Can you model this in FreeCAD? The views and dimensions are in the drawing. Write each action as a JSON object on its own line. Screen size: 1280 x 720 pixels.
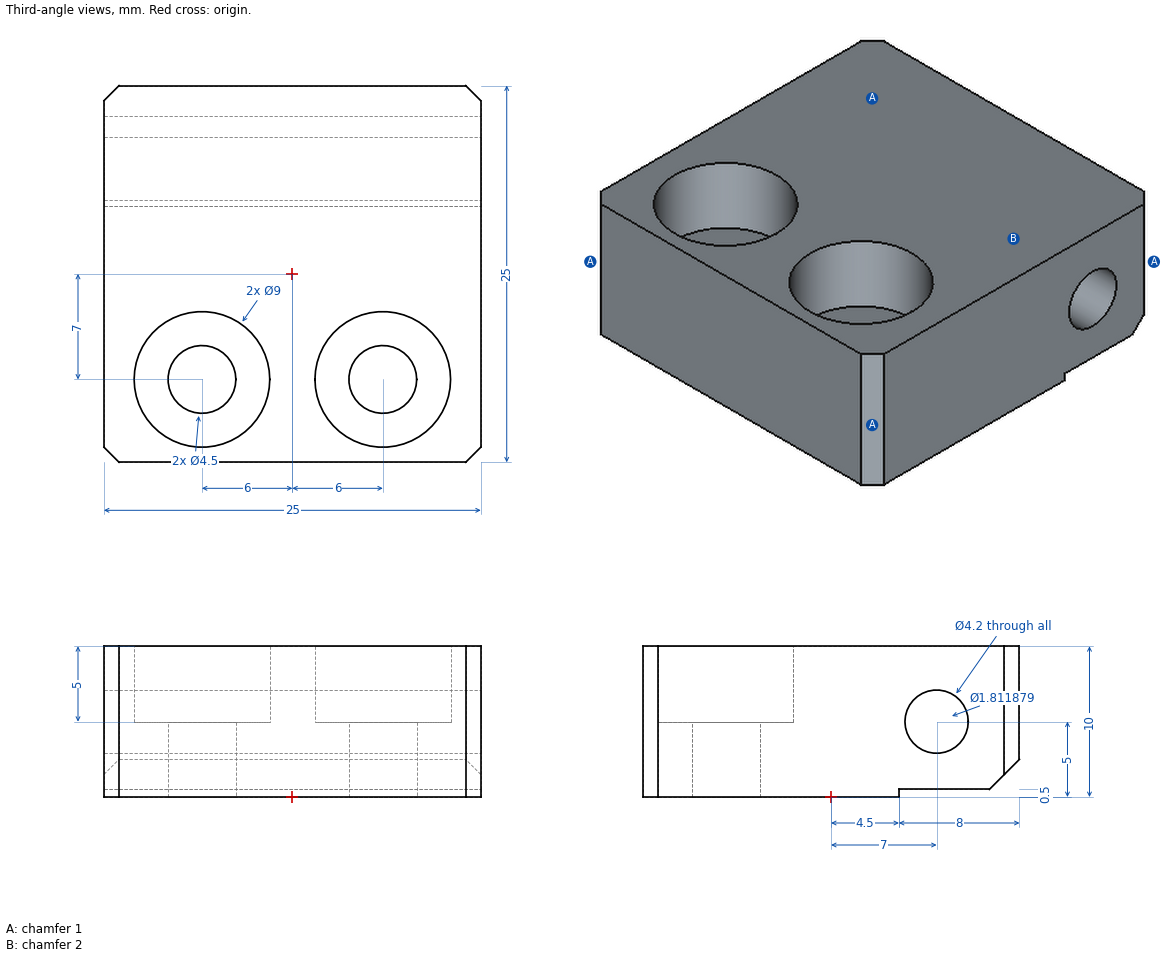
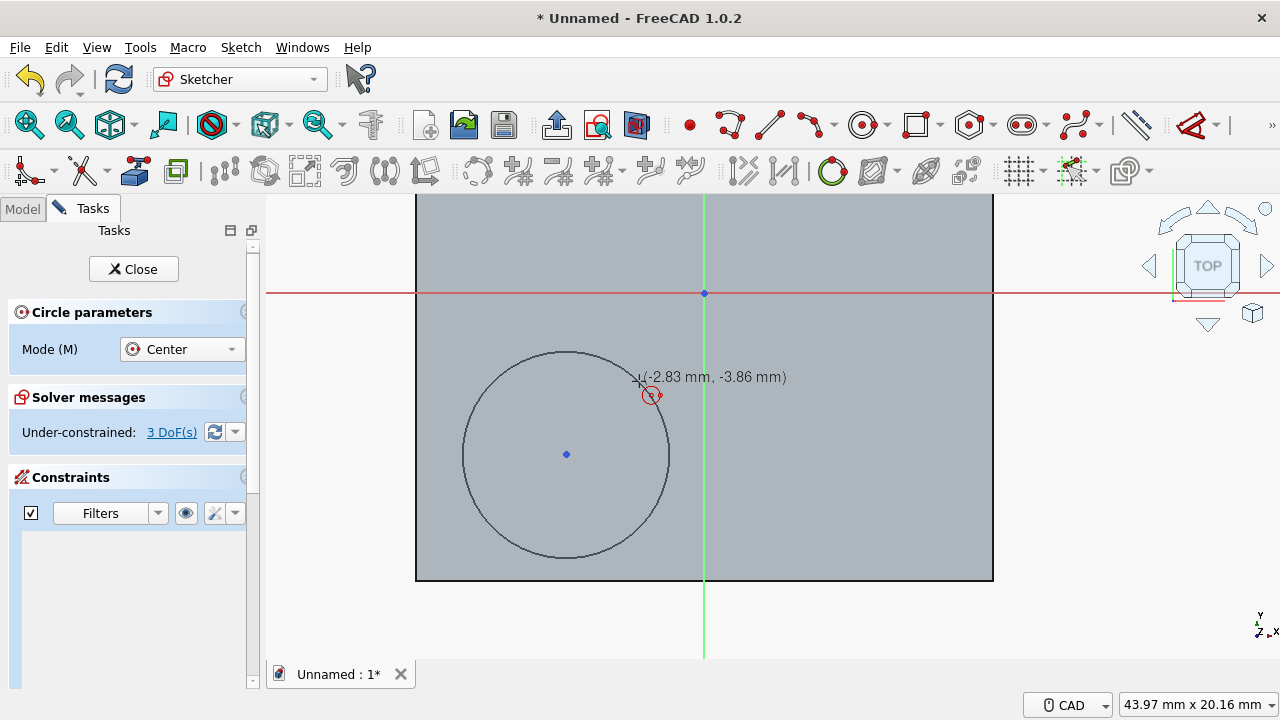
{"action": "left_click", "coordinate": [843, 454]}
{"action": "left_click", "coordinate": [916, 381]}
{"action": "key", "text": "Escape"}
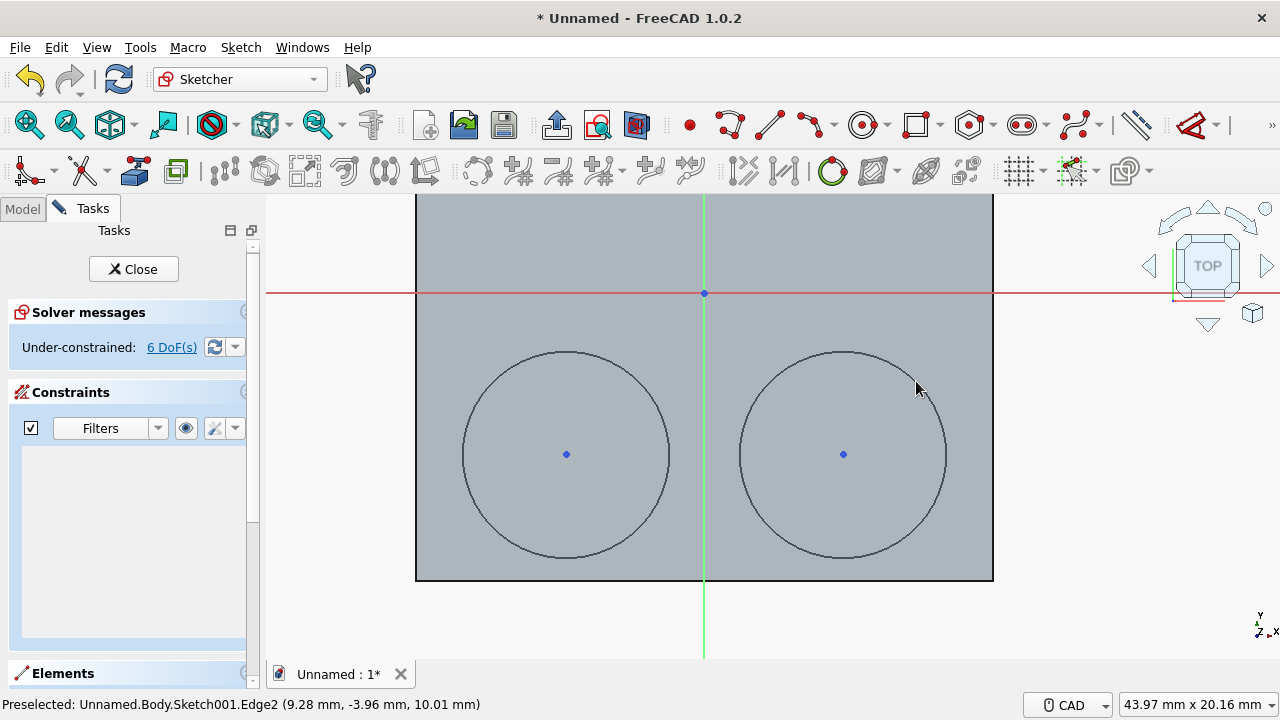
{"action": "left_click", "coordinate": [639, 382]}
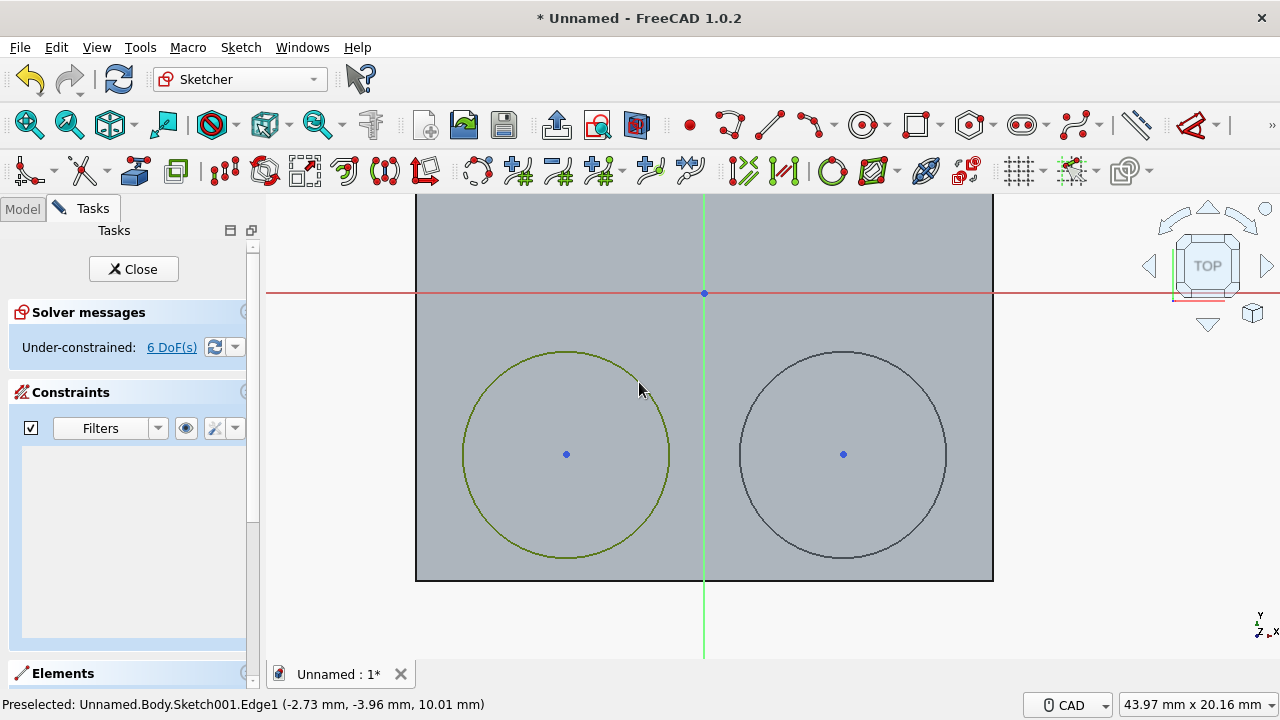
{"action": "left_click", "coordinate": [916, 382]}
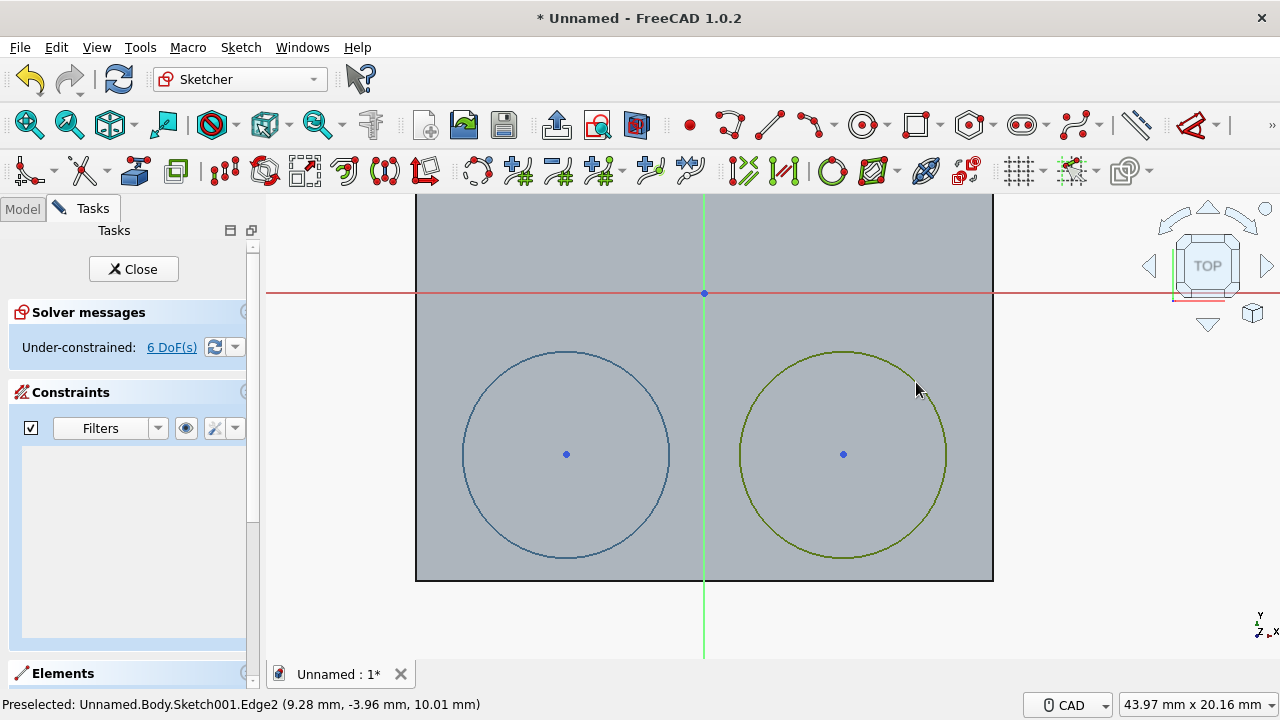
{"action": "key", "text": "e"}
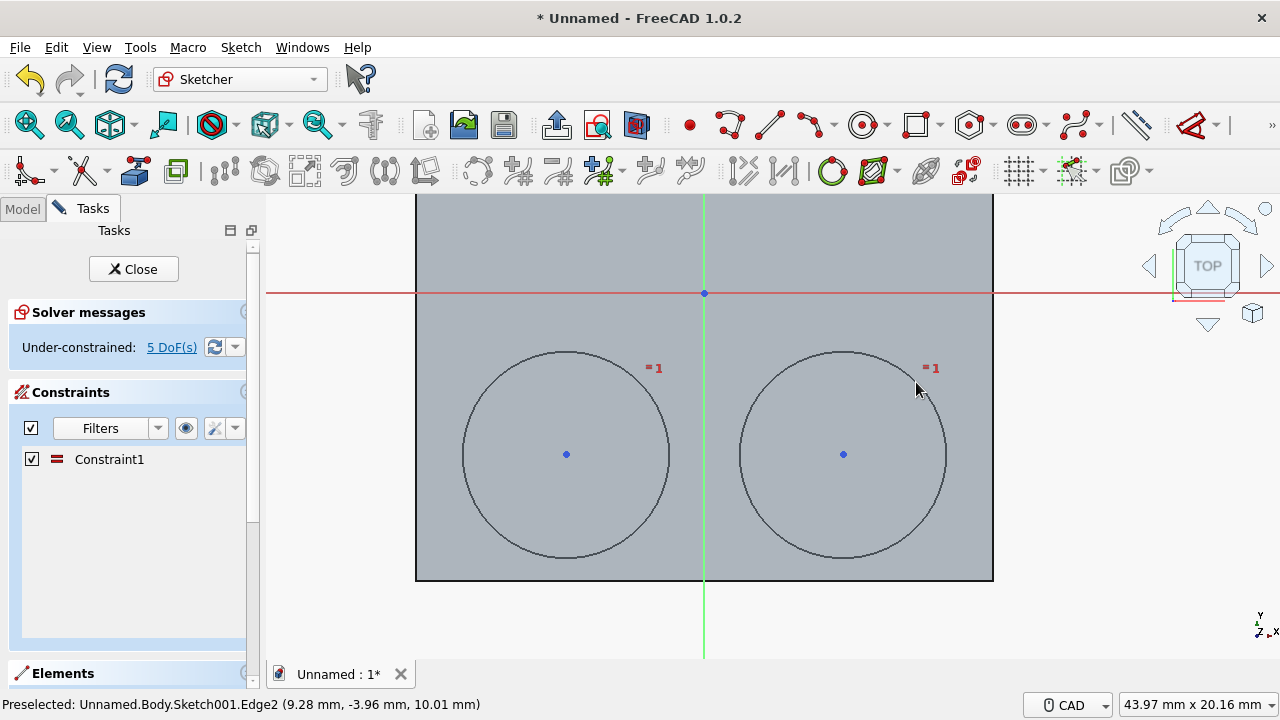
{"action": "left_click", "coordinate": [566, 455]}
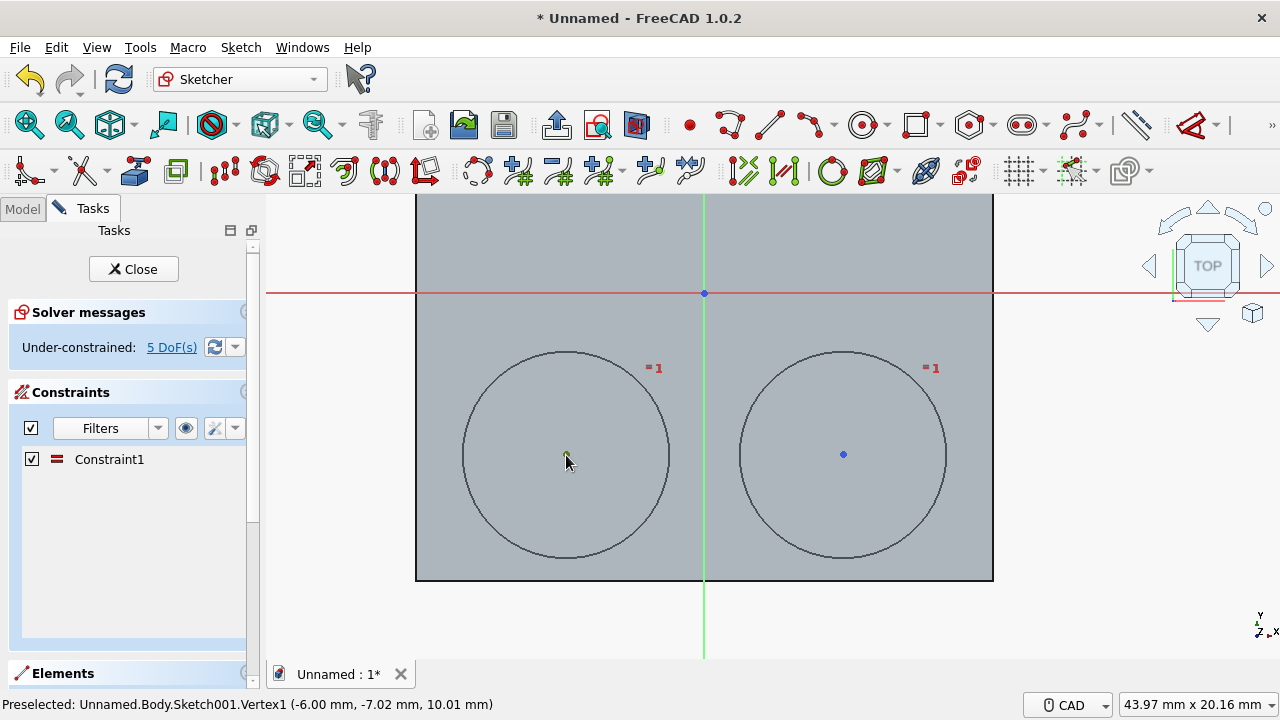
{"action": "left_click", "coordinate": [843, 455]}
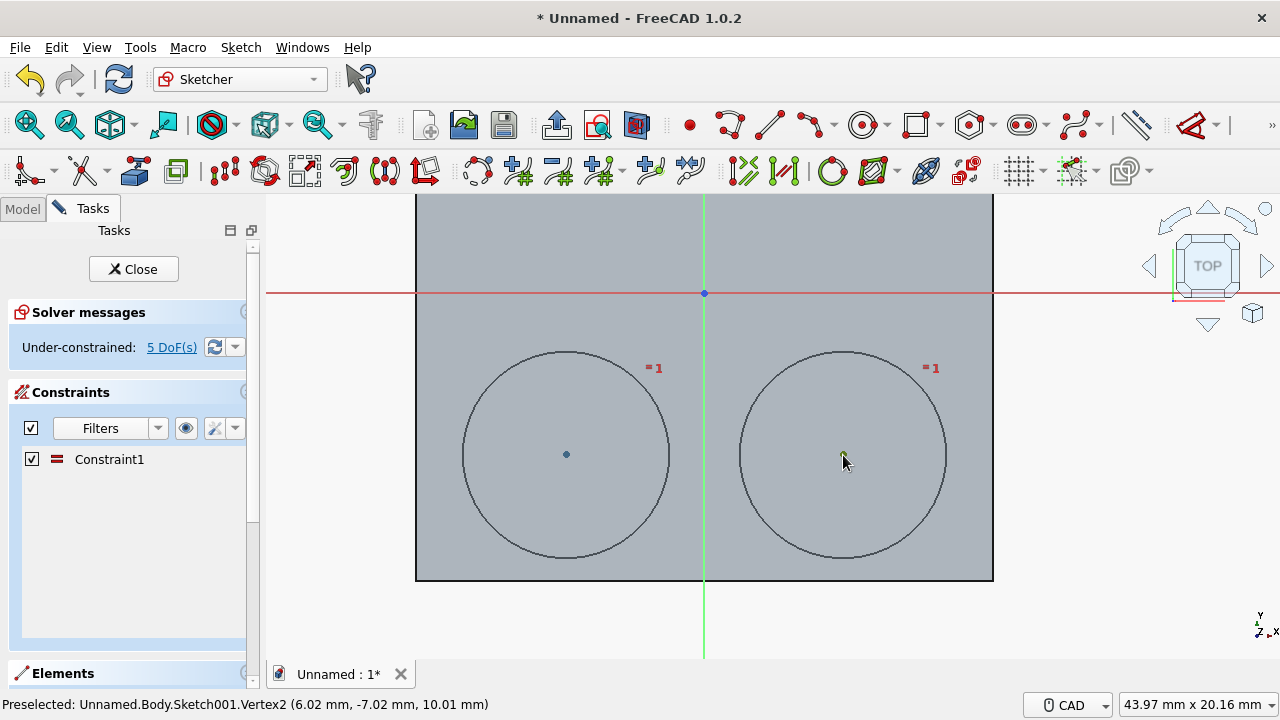
{"action": "key", "text": "h"}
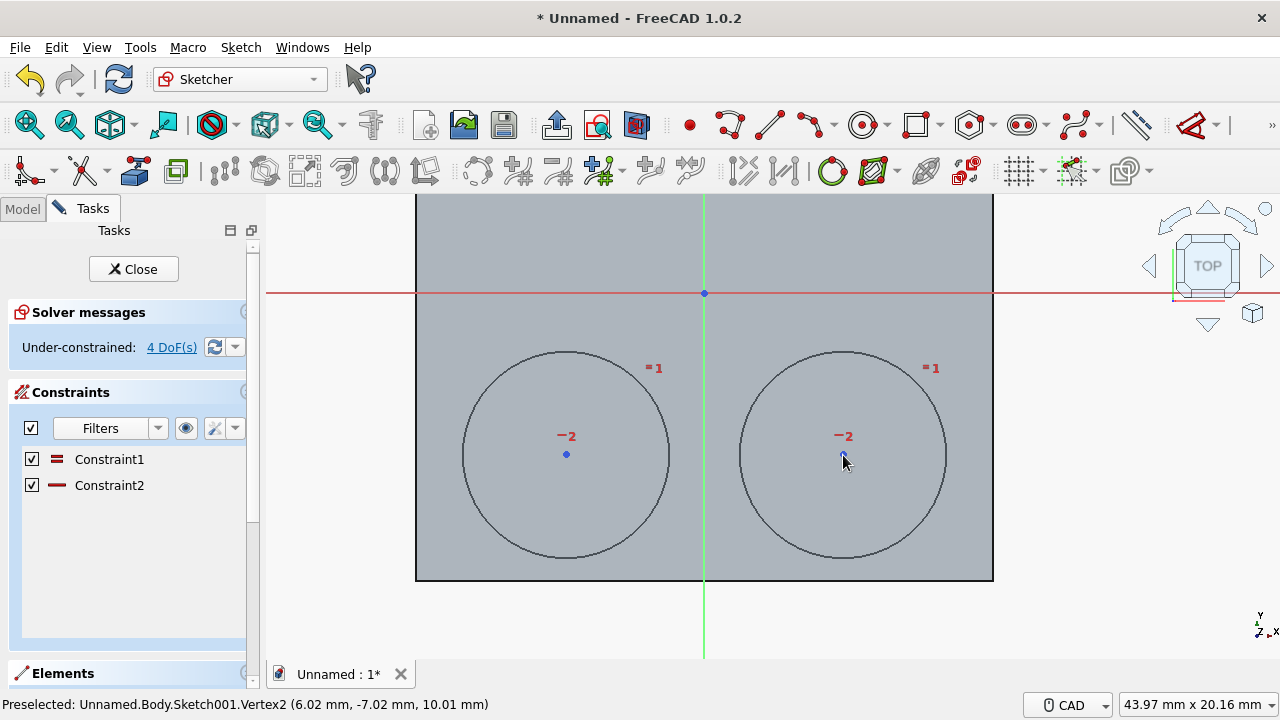
{"action": "left_click", "coordinate": [1192, 126]}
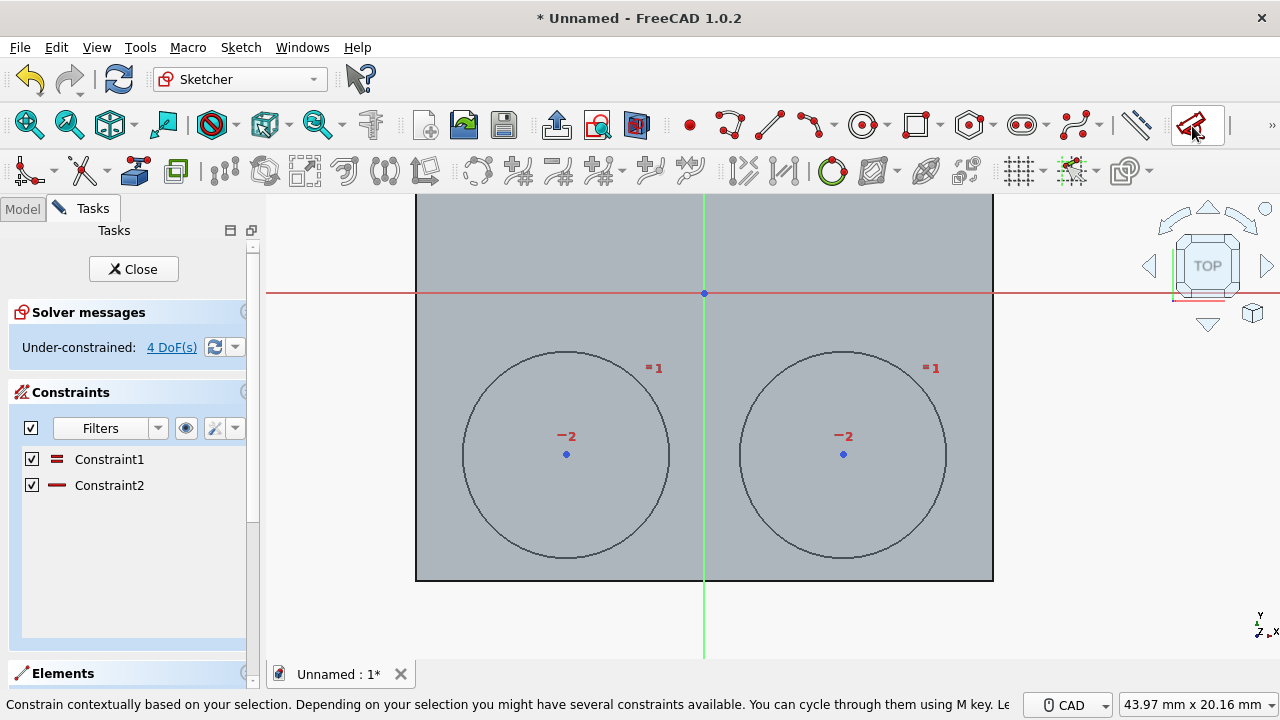
{"action": "left_click", "coordinate": [639, 382]}
{"action": "left_click", "coordinate": [662, 359]}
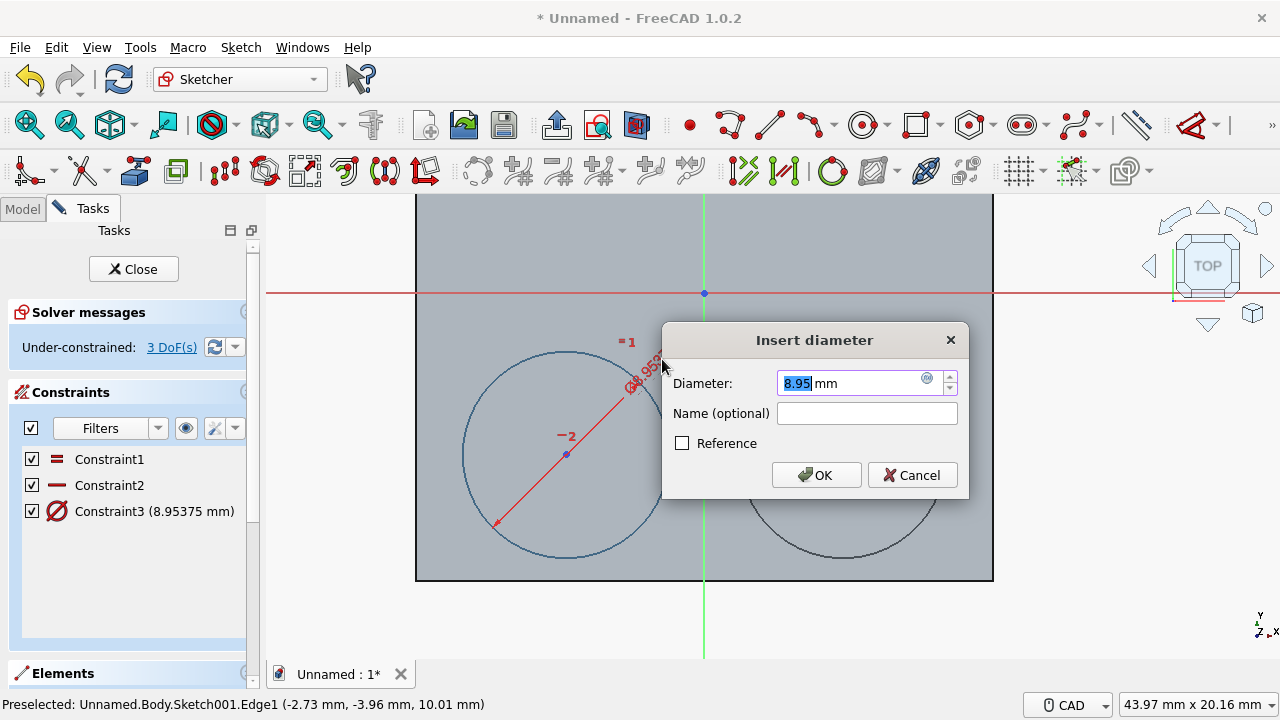
{"action": "type", "text": "9"}
{"action": "key", "text": "Return"}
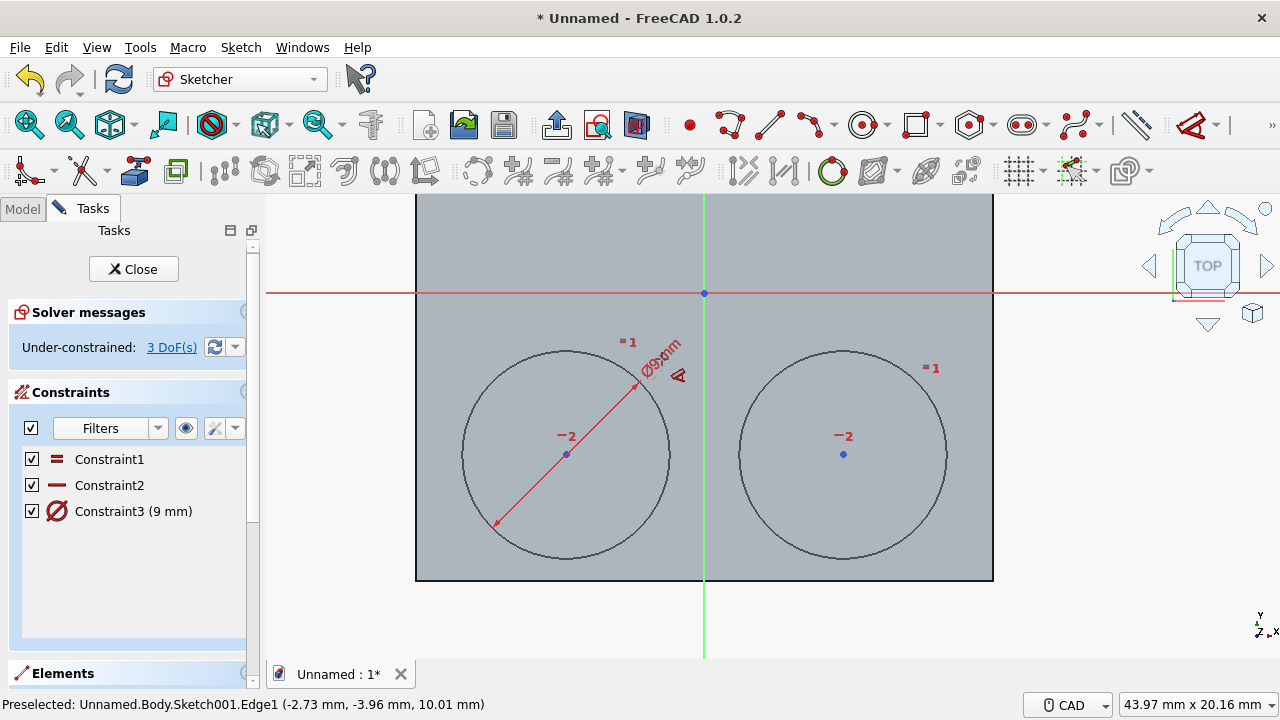
{"action": "left_click", "coordinate": [566, 455]}
{"action": "left_click", "coordinate": [635, 259]}